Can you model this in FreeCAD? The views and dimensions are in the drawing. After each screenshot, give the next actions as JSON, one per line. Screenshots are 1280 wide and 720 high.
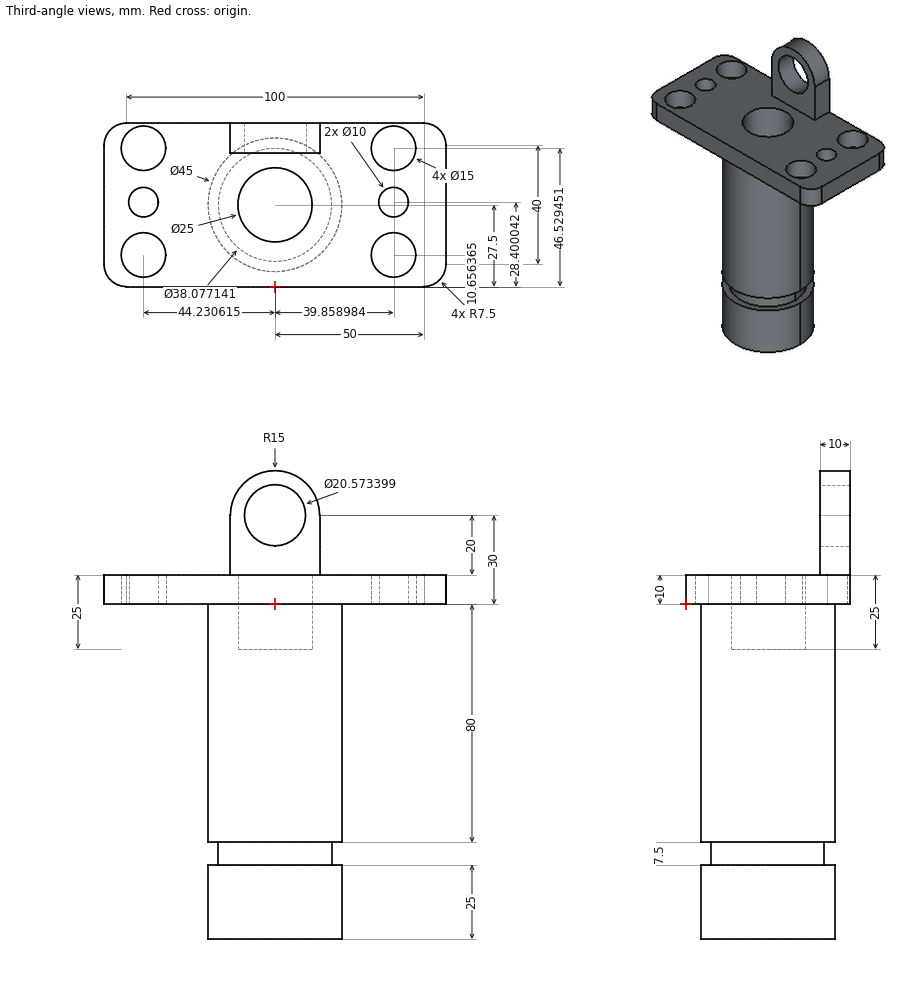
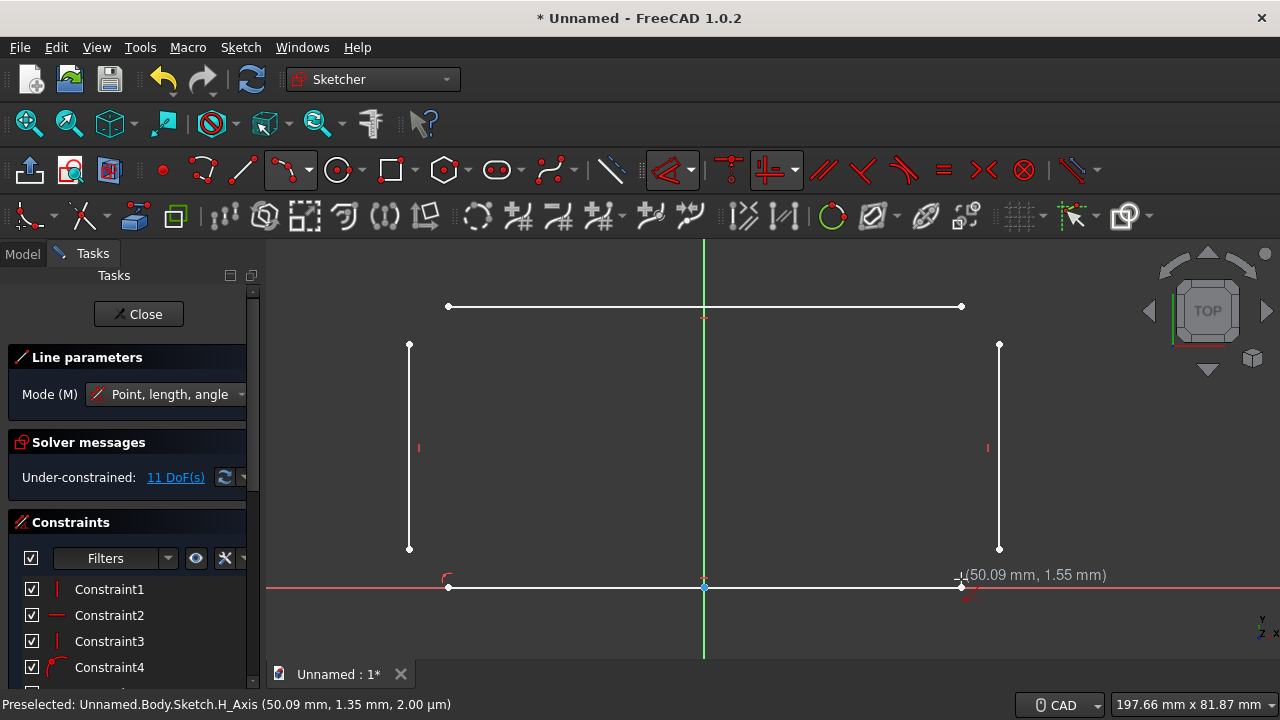
{"action": "left_click", "coordinate": [284, 170]}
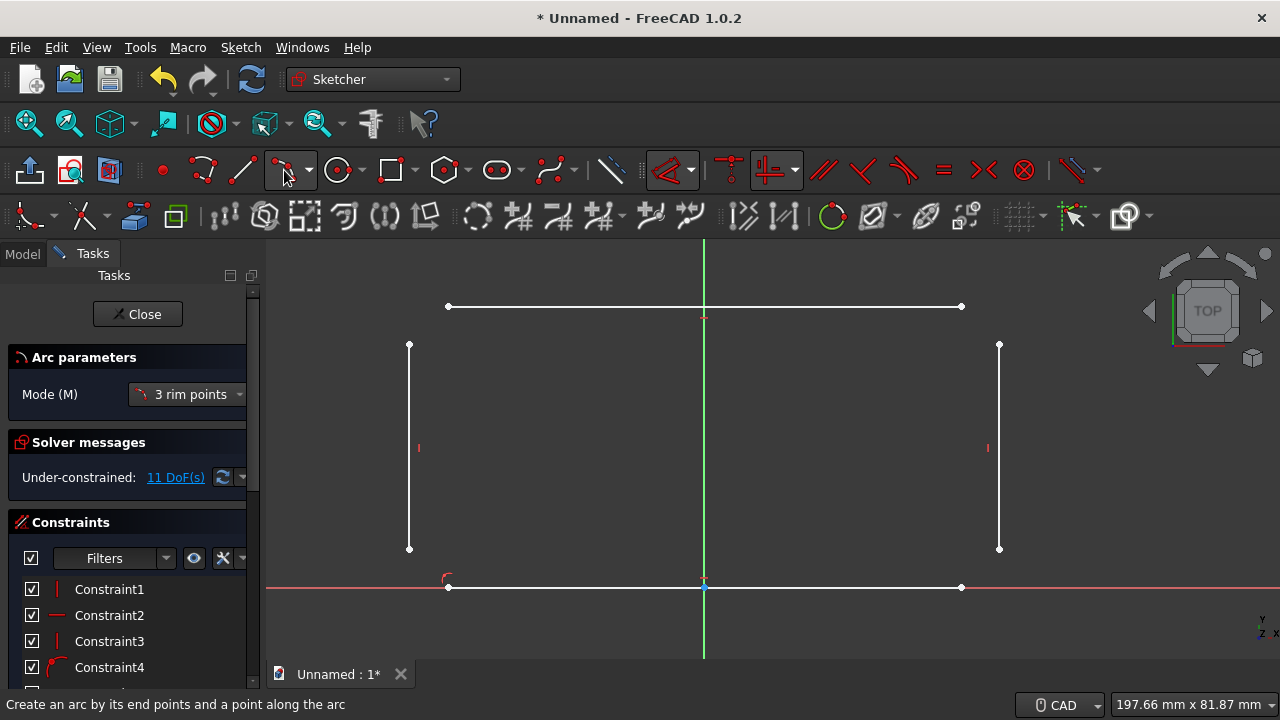
{"action": "left_click", "coordinate": [999, 345]}
{"action": "left_click", "coordinate": [961, 307]}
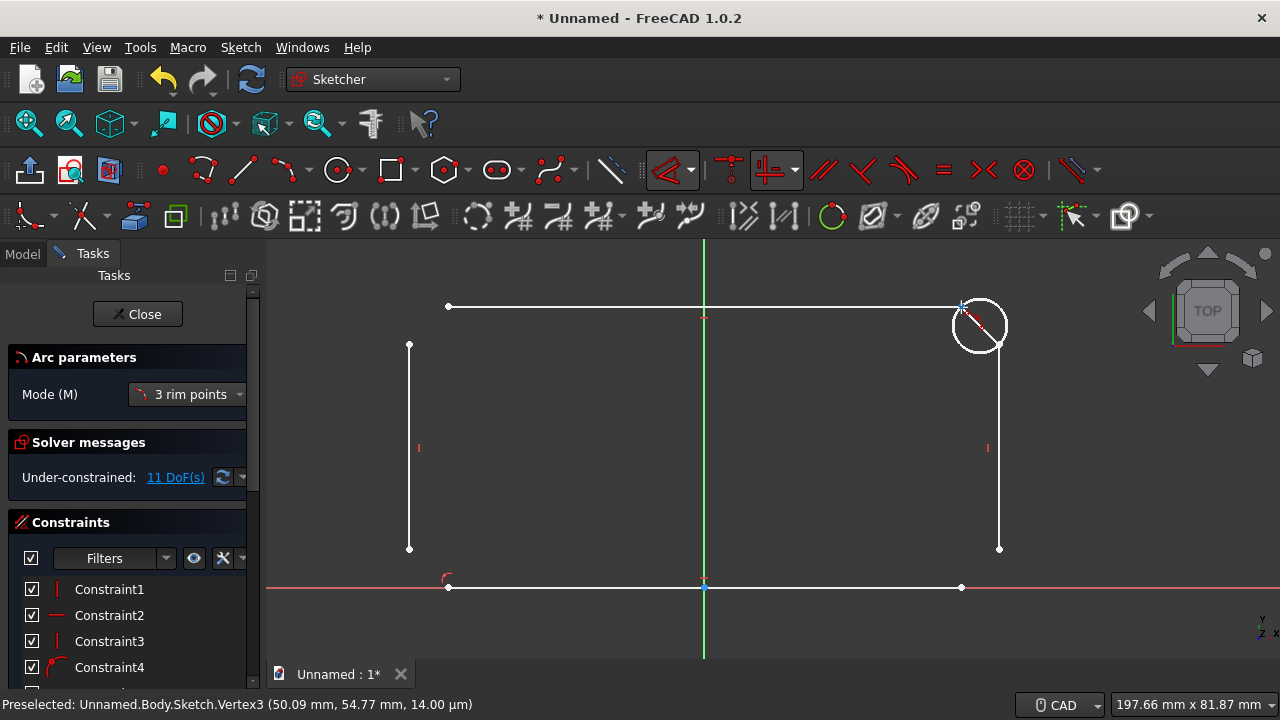
{"action": "scroll", "coordinate": [988, 317], "scroll_direction": "up", "scroll_amount": 2}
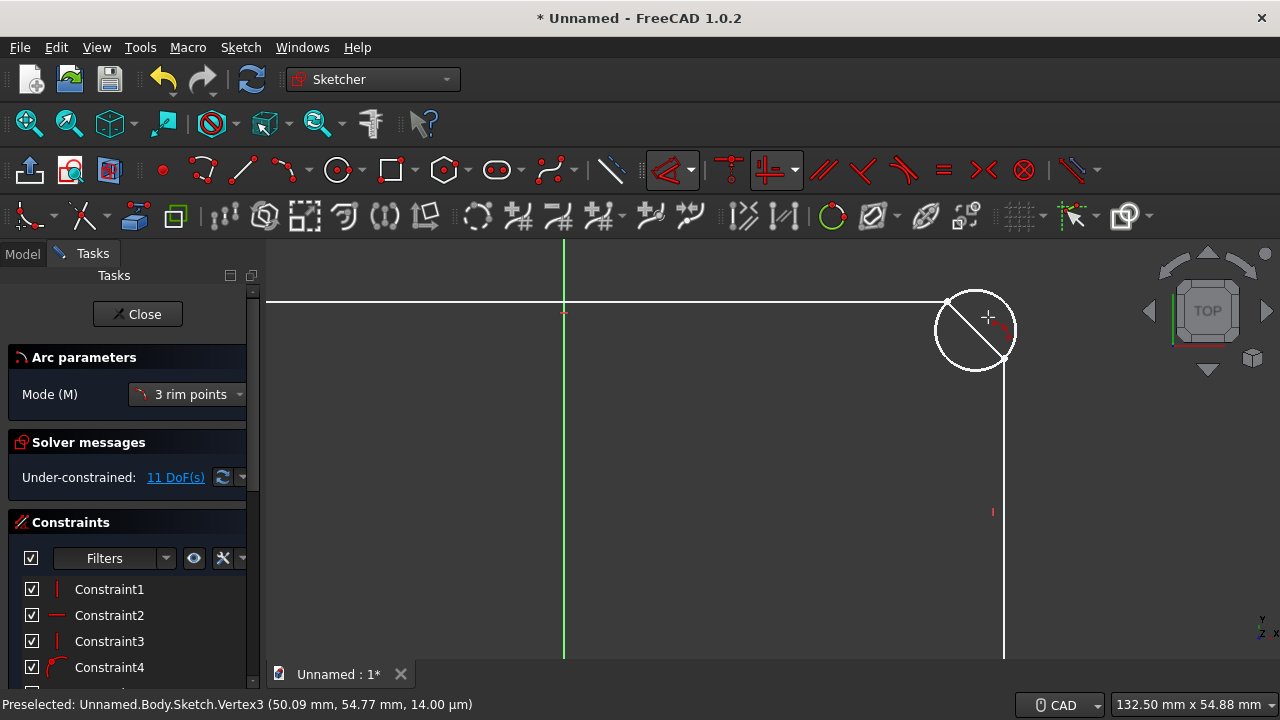
{"action": "left_click", "coordinate": [987, 317]}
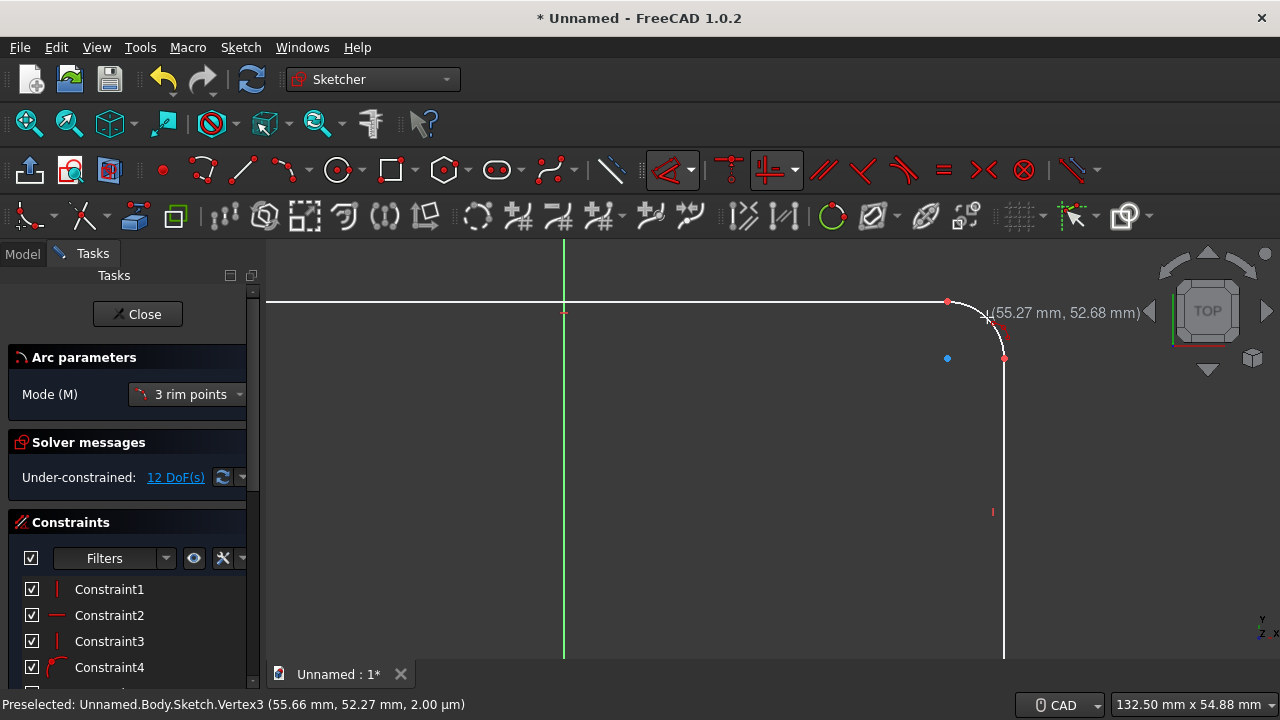
{"action": "scroll", "coordinate": [990, 324], "scroll_direction": "down", "scroll_amount": 2}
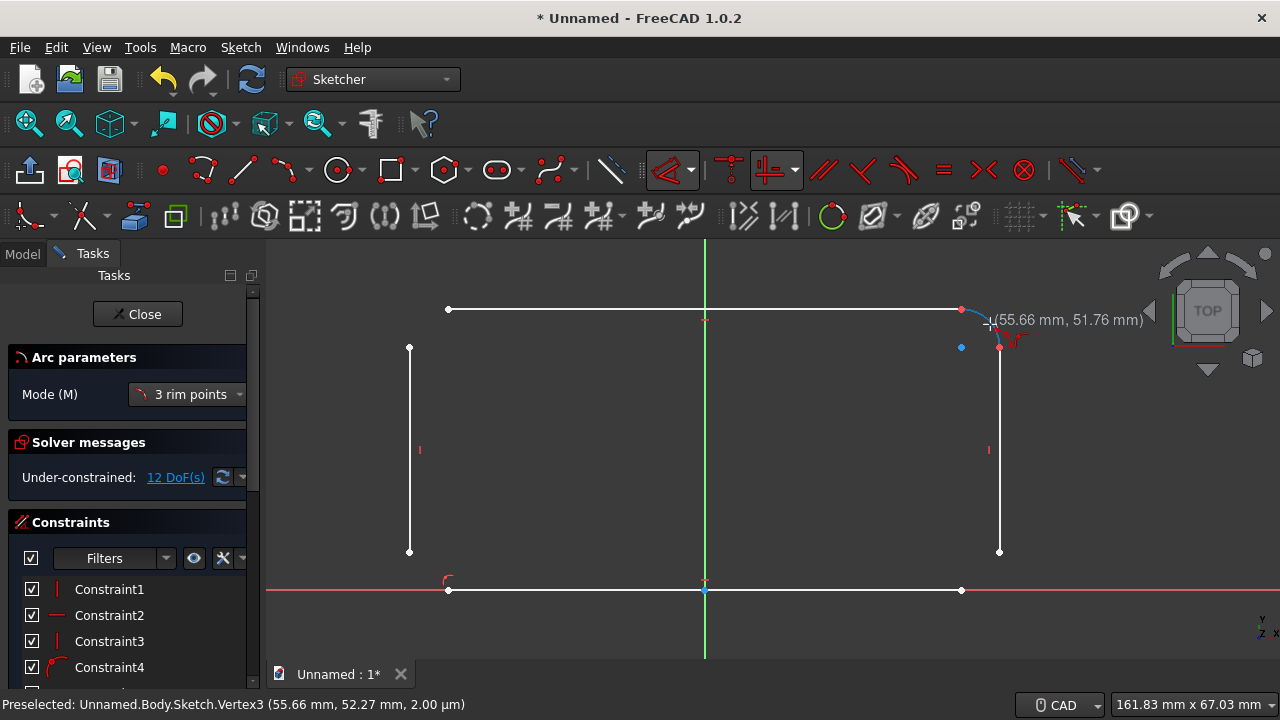
{"action": "left_click", "coordinate": [449, 309]}
{"action": "left_click", "coordinate": [410, 347]}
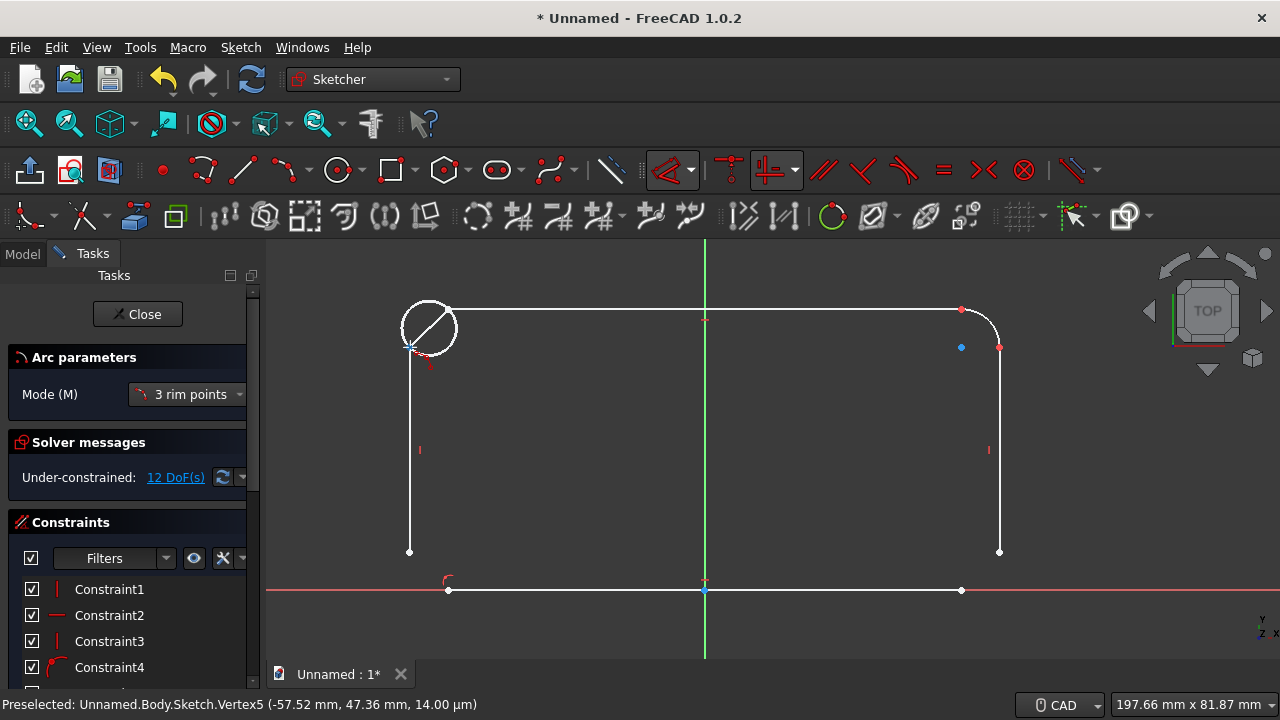
{"action": "scroll", "coordinate": [421, 319], "scroll_direction": "up", "scroll_amount": 2}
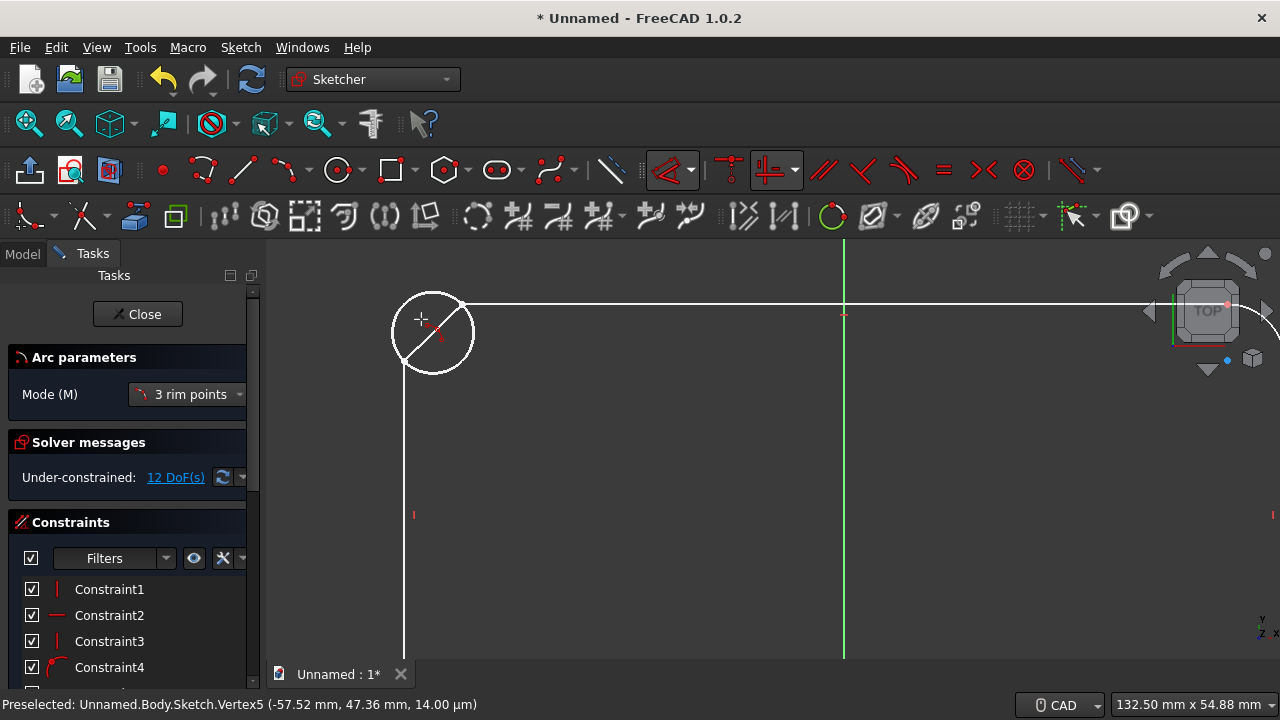
{"action": "left_click", "coordinate": [421, 319]}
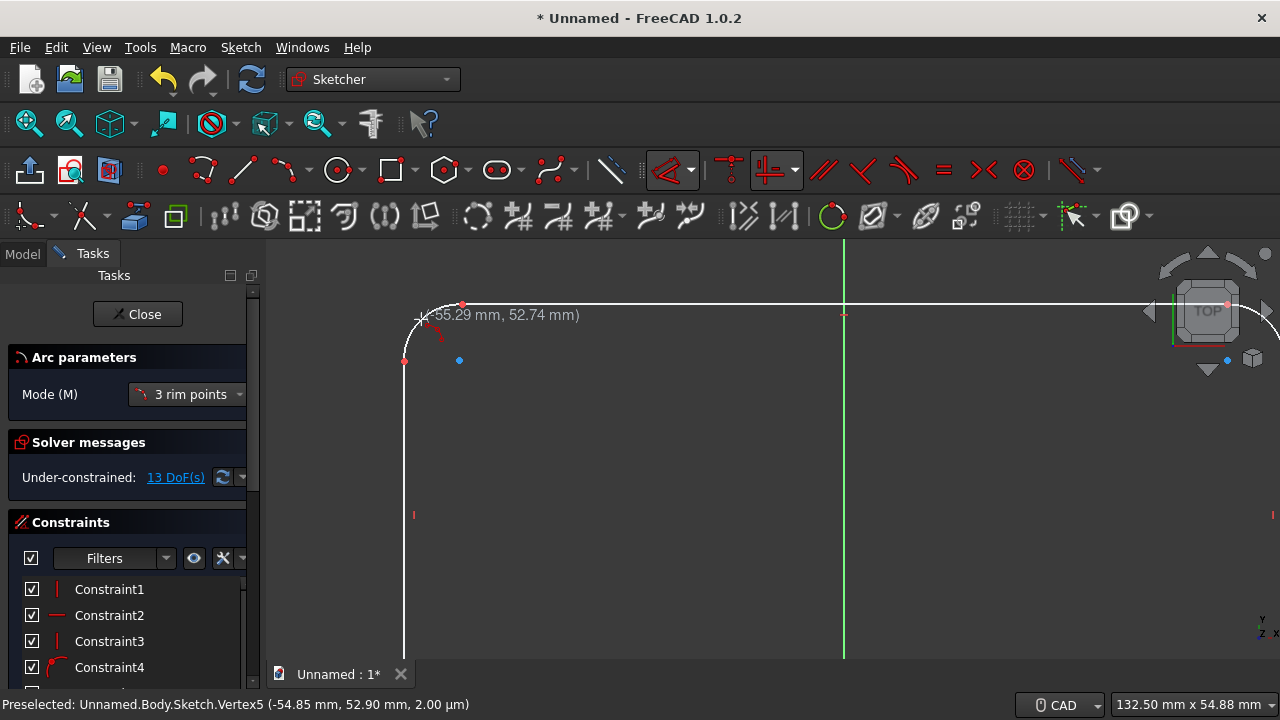
{"action": "scroll", "coordinate": [421, 319], "scroll_direction": "down", "scroll_amount": 2}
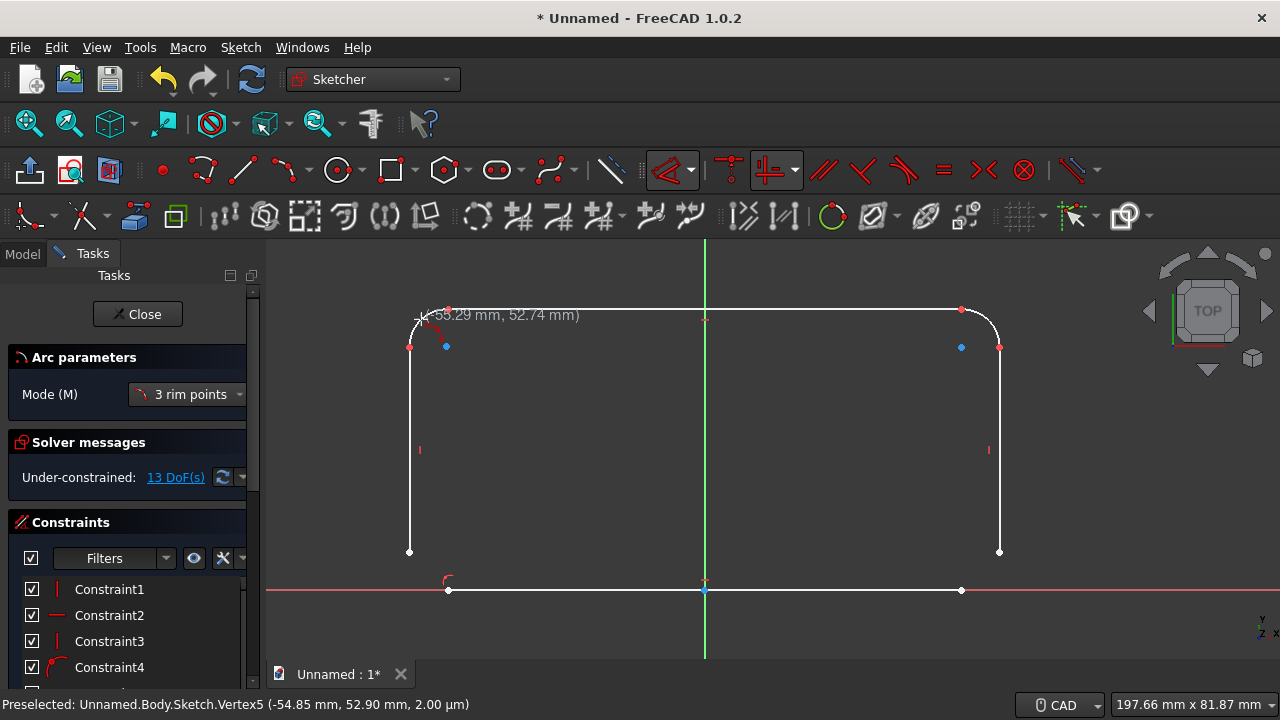
{"action": "left_click", "coordinate": [410, 552]}
{"action": "left_click", "coordinate": [449, 590]}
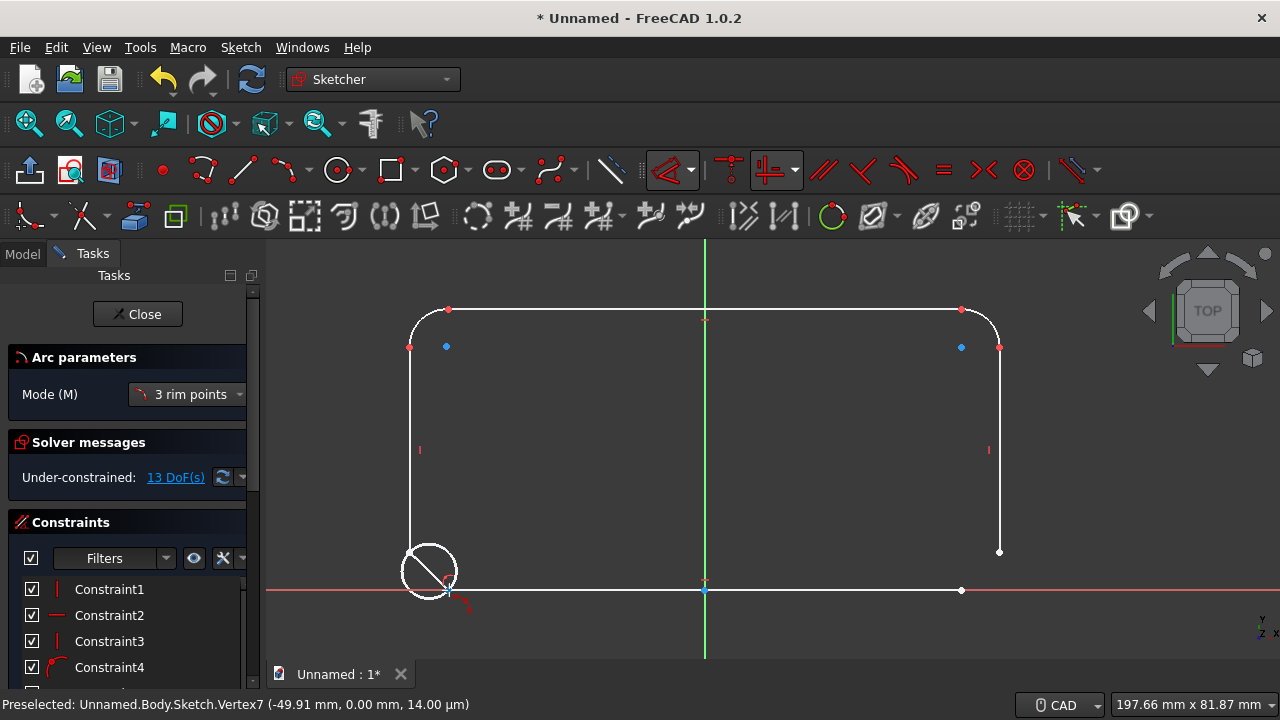
{"action": "scroll", "coordinate": [421, 579], "scroll_direction": "up", "scroll_amount": 2}